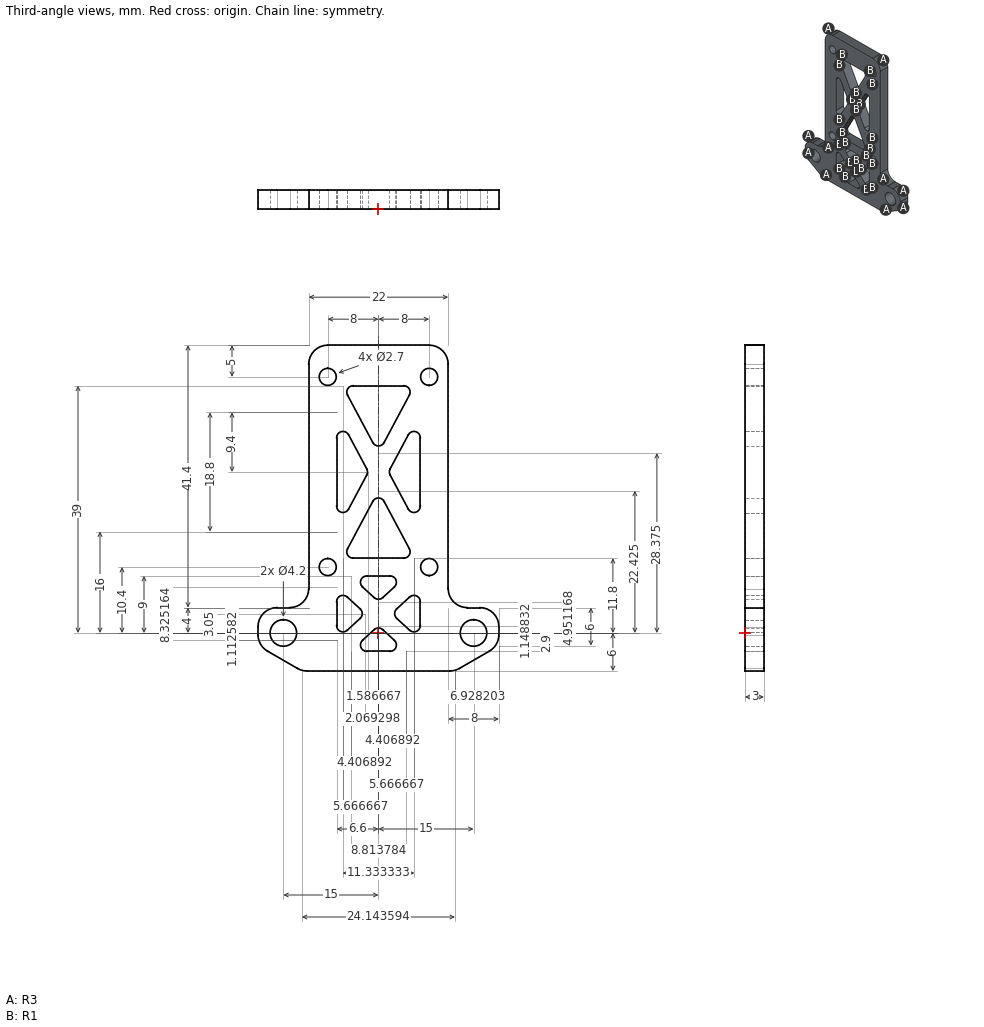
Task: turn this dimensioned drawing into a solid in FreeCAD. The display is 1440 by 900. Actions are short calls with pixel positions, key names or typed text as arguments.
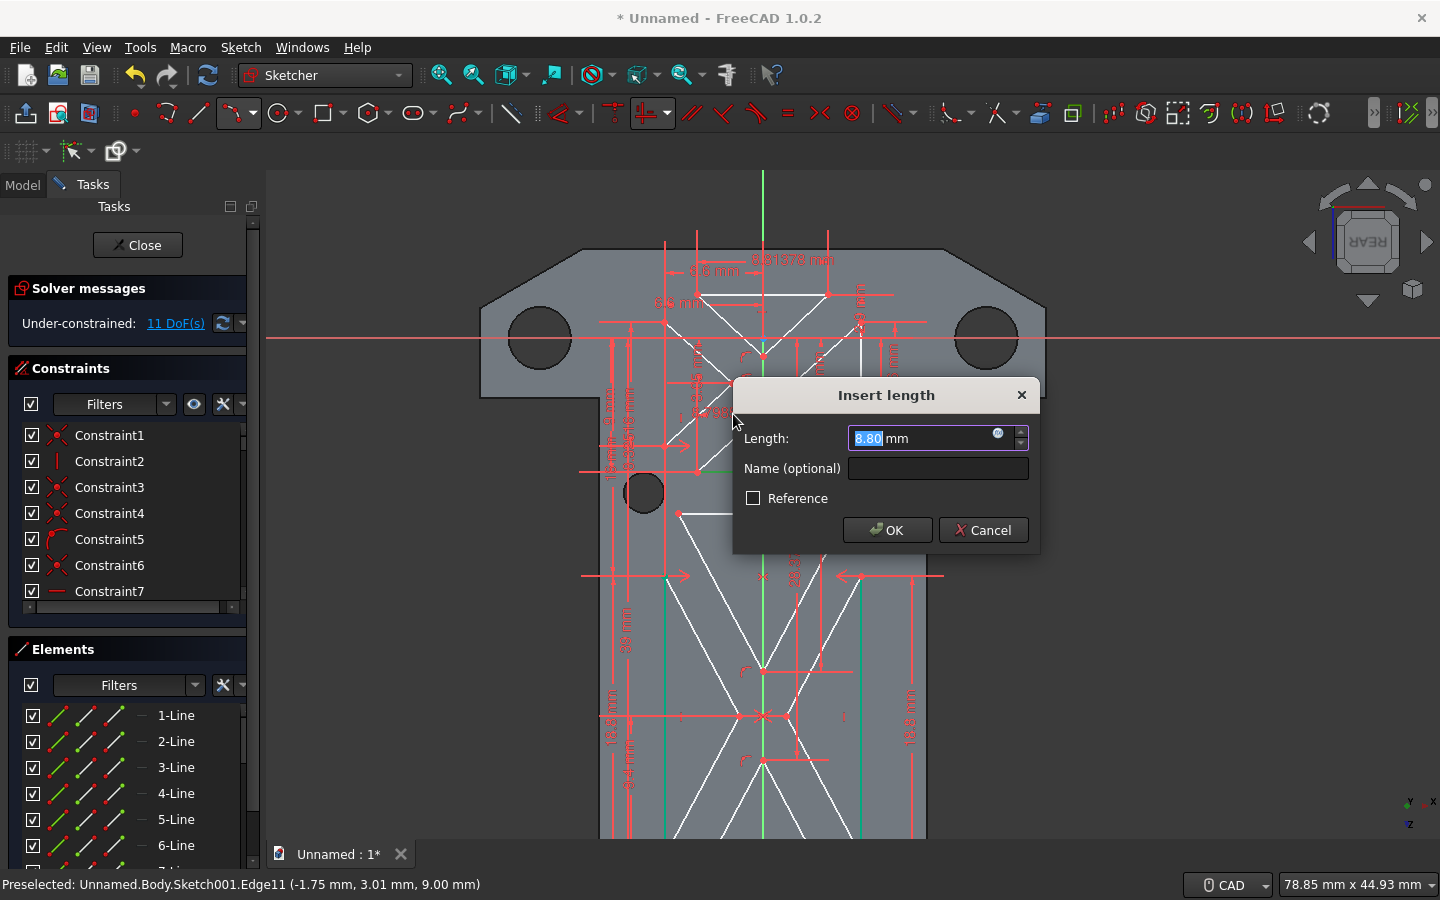
text(8.813784)
key(Return)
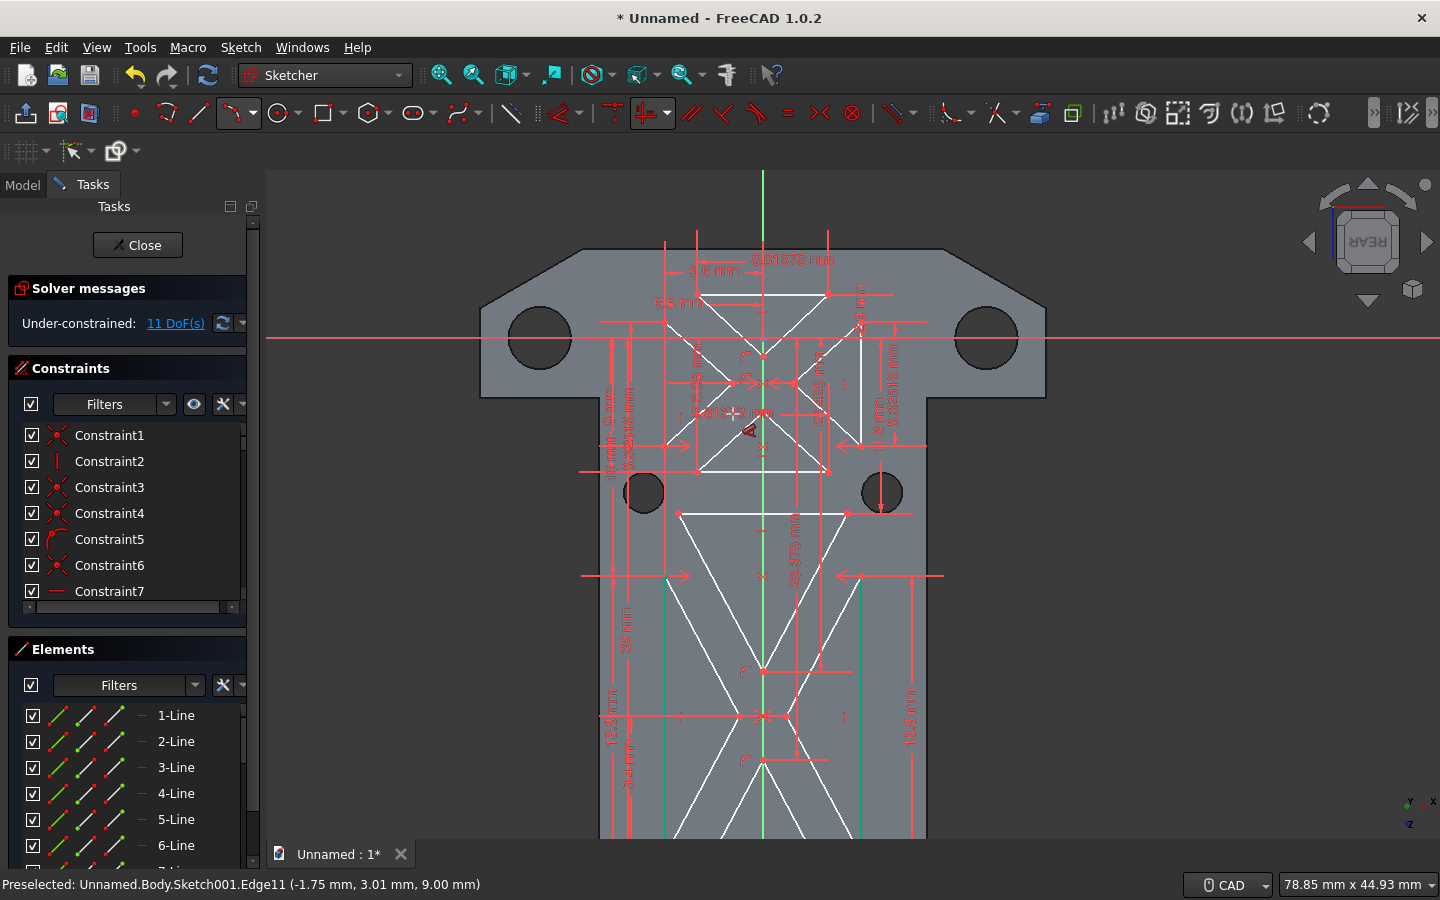
click(797, 514)
click(724, 548)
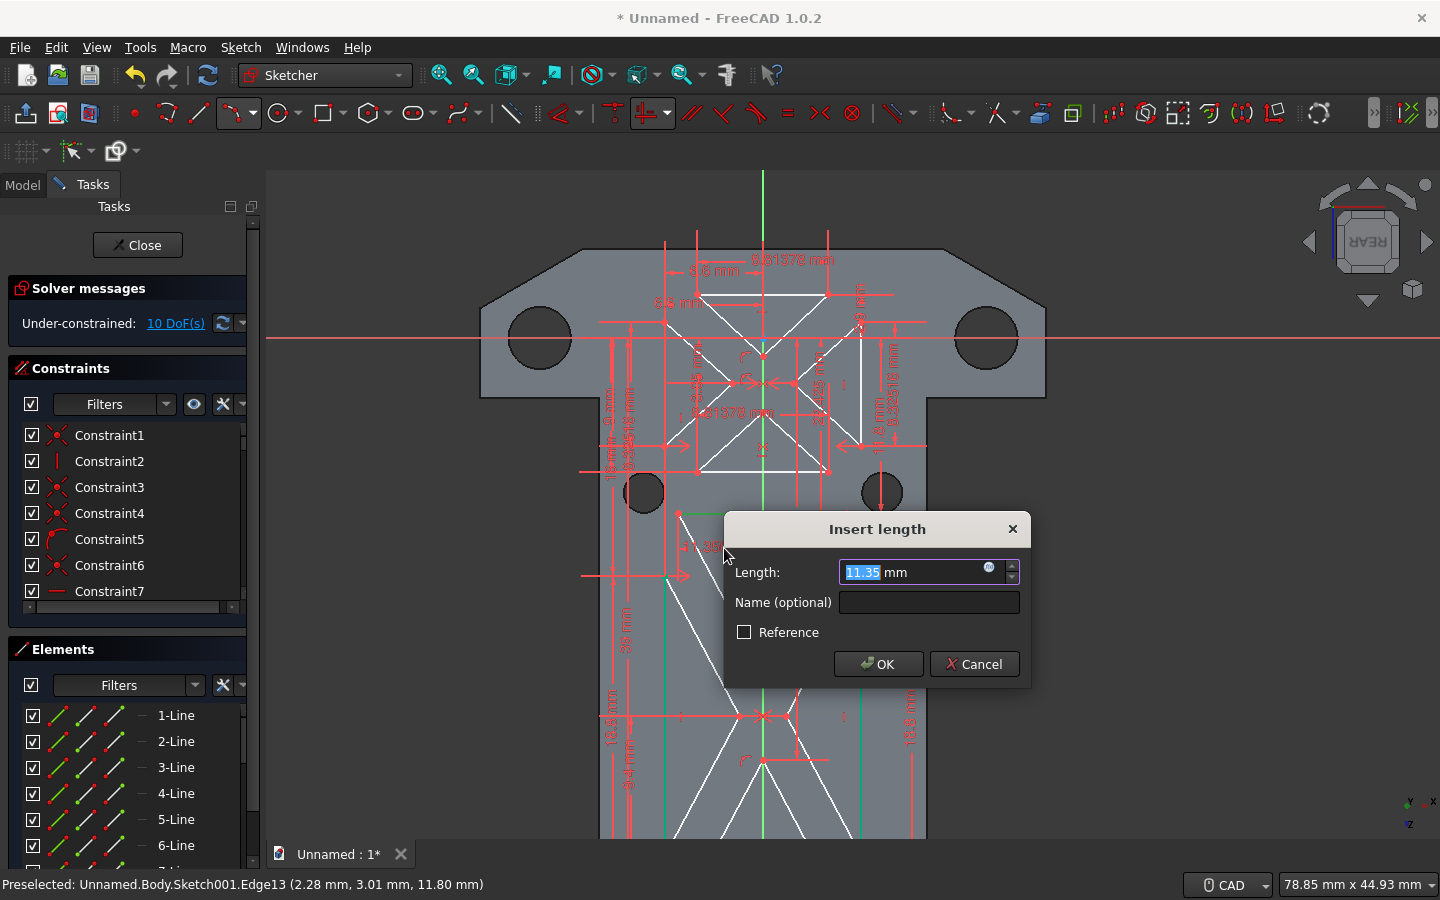
text(11.333333)
key(Return)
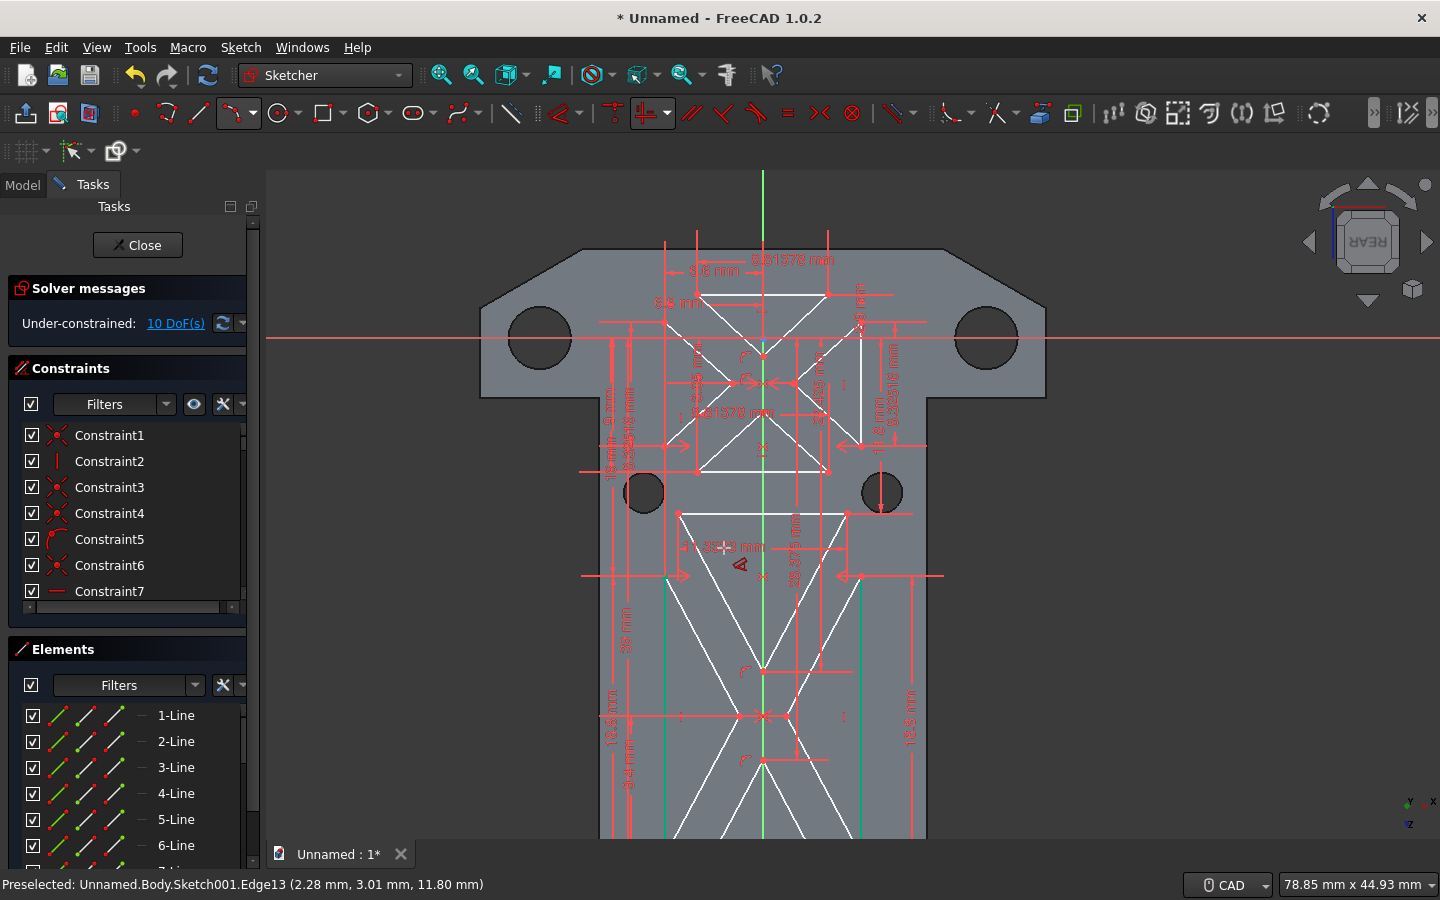
scroll(828, 297, down, 2)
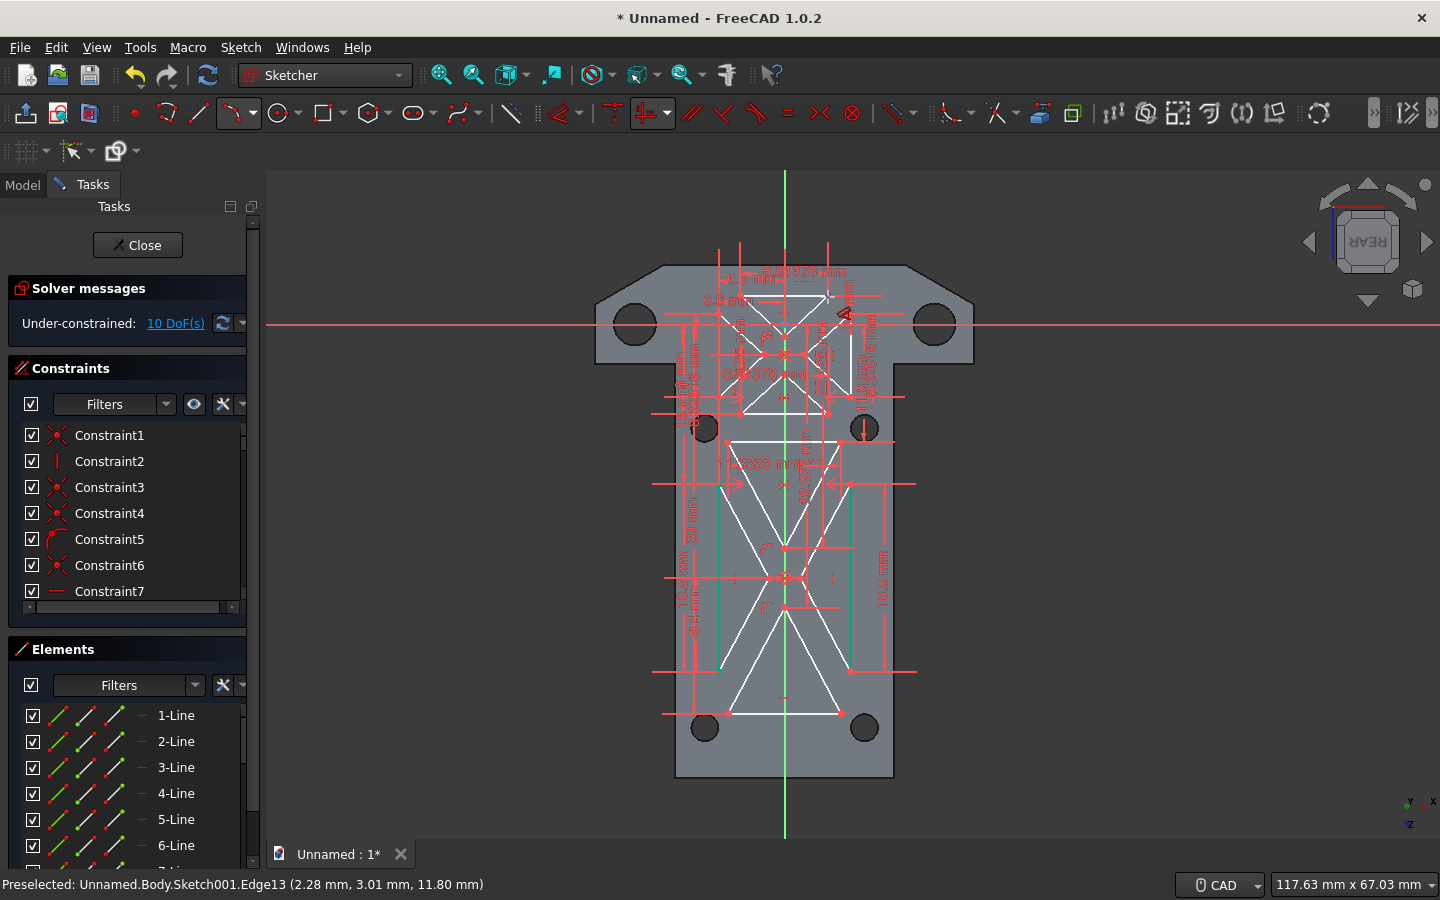
click(762, 714)
click(759, 748)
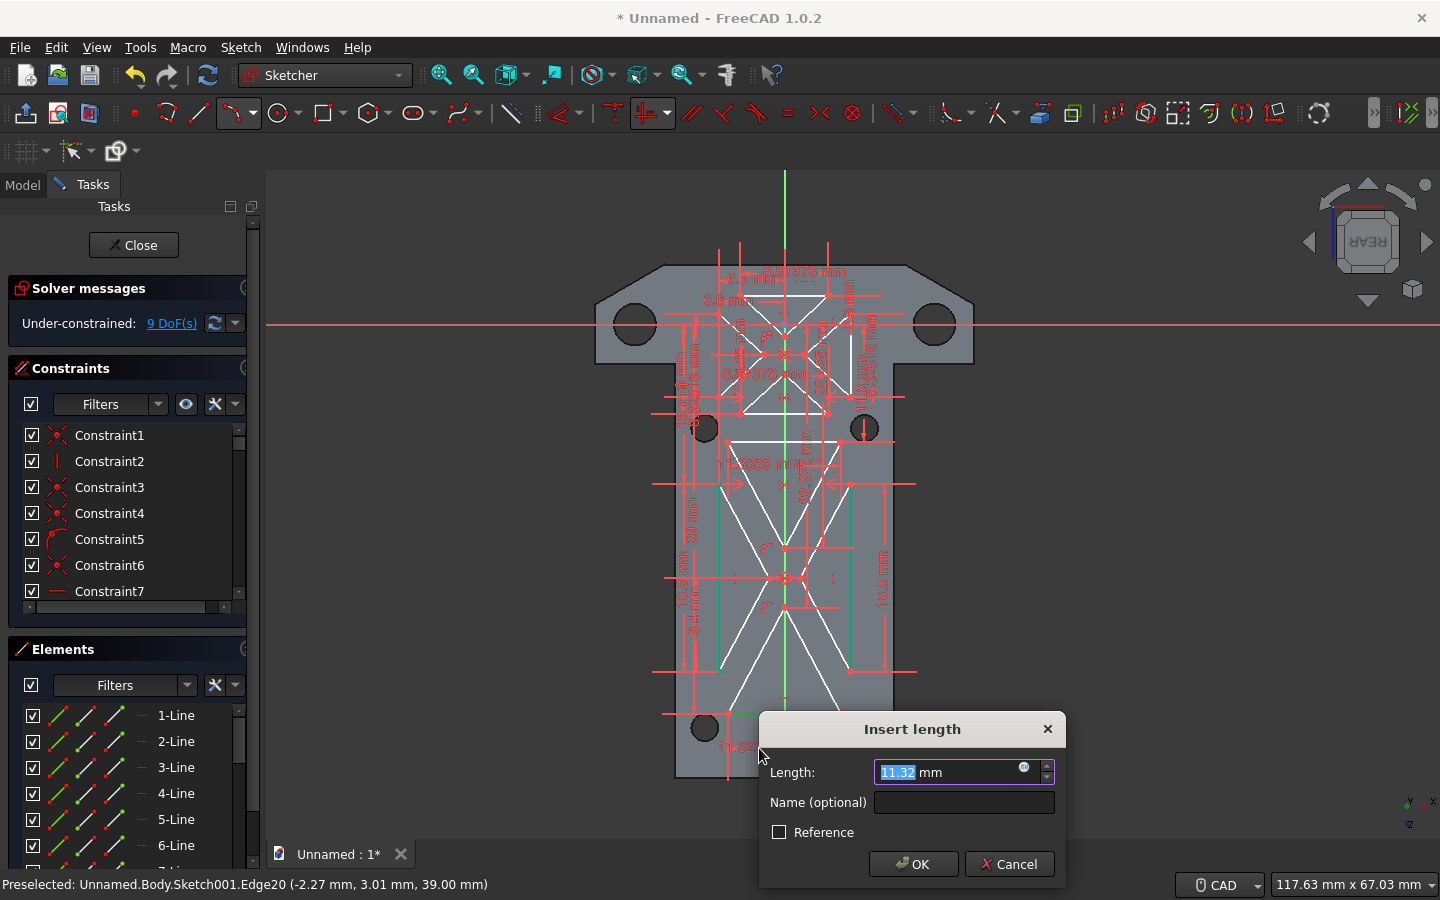
text(11.333333)
key(Return)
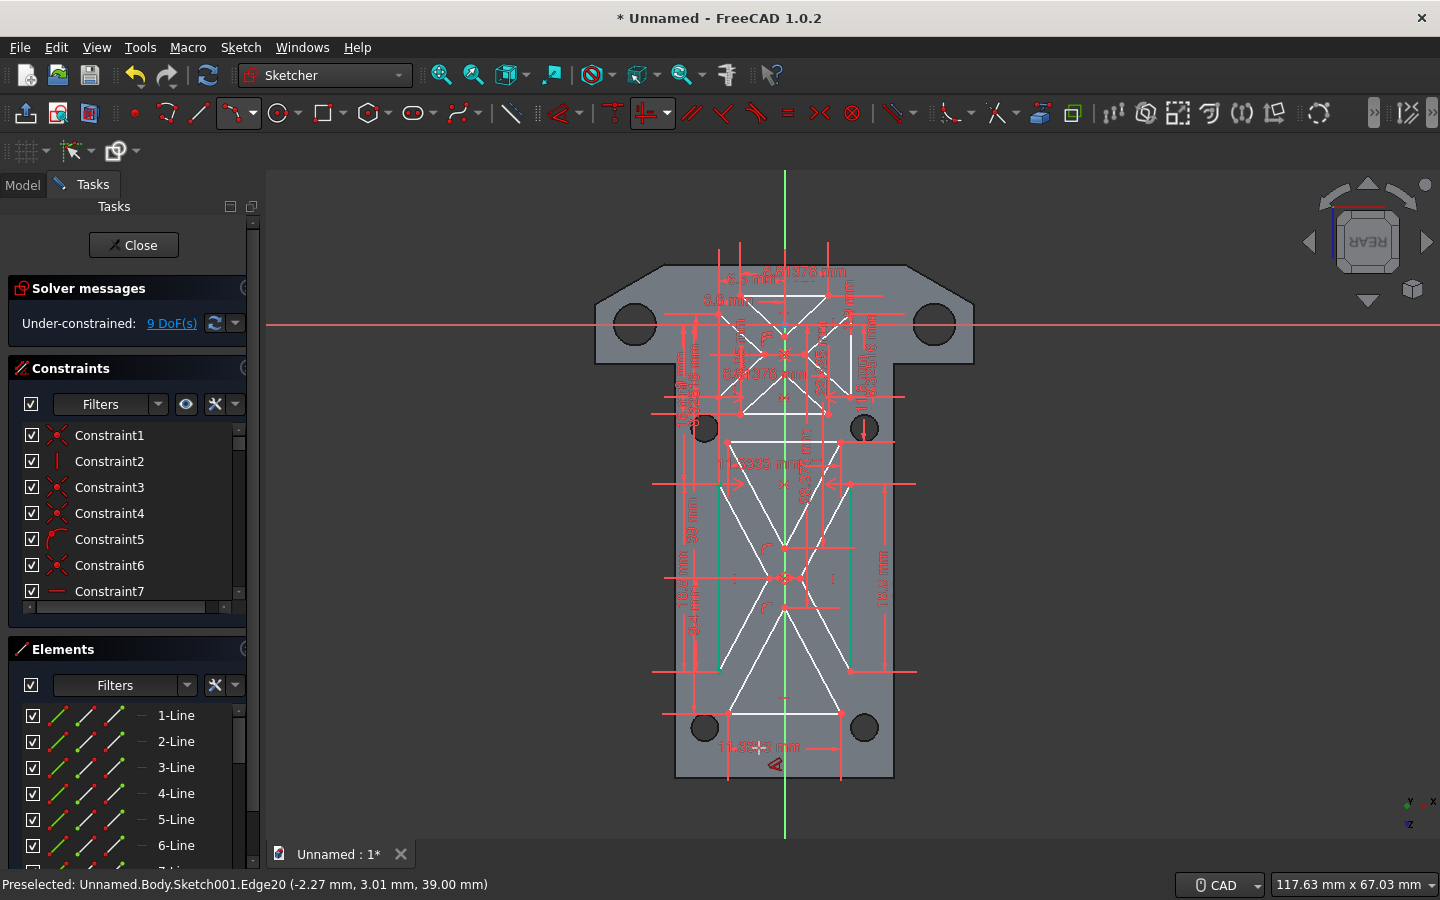
scroll(764, 355, up, 4)